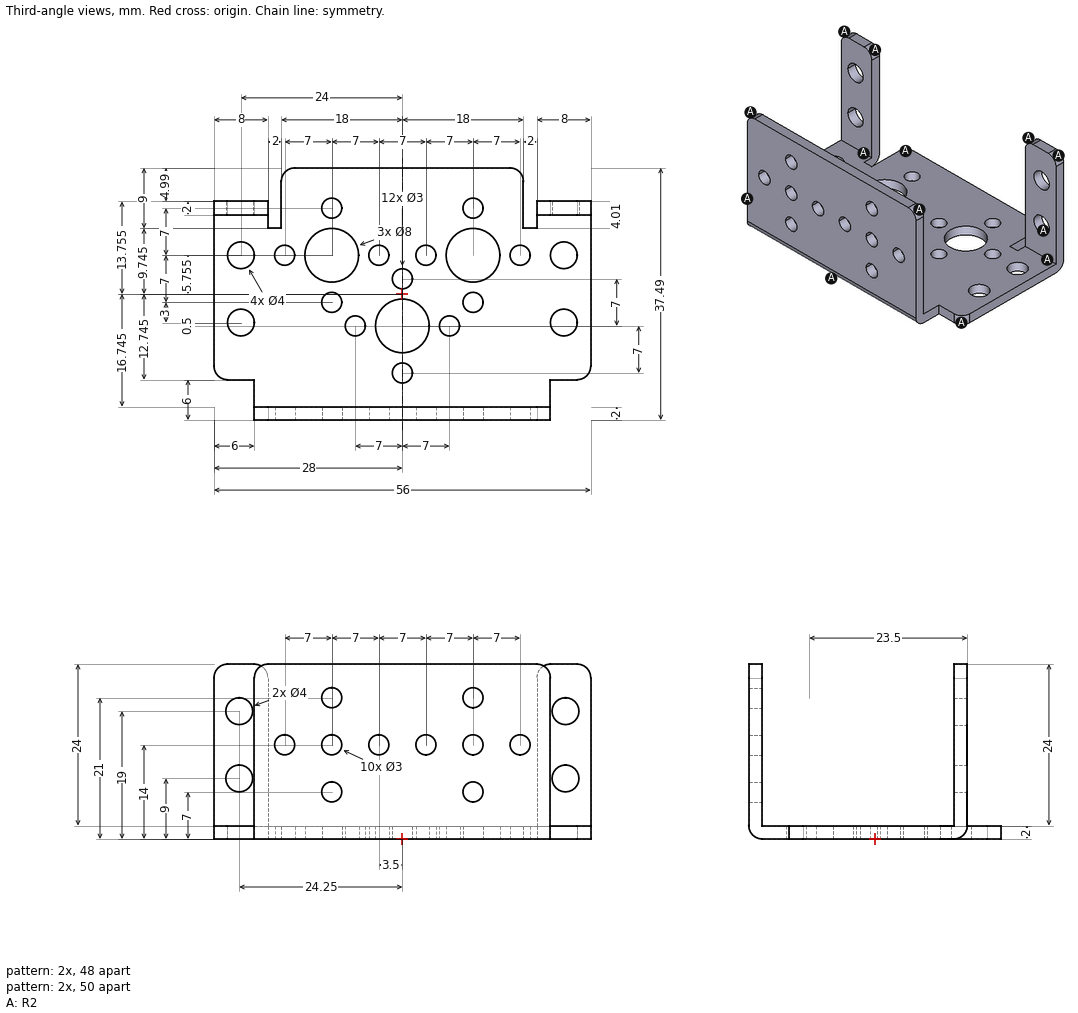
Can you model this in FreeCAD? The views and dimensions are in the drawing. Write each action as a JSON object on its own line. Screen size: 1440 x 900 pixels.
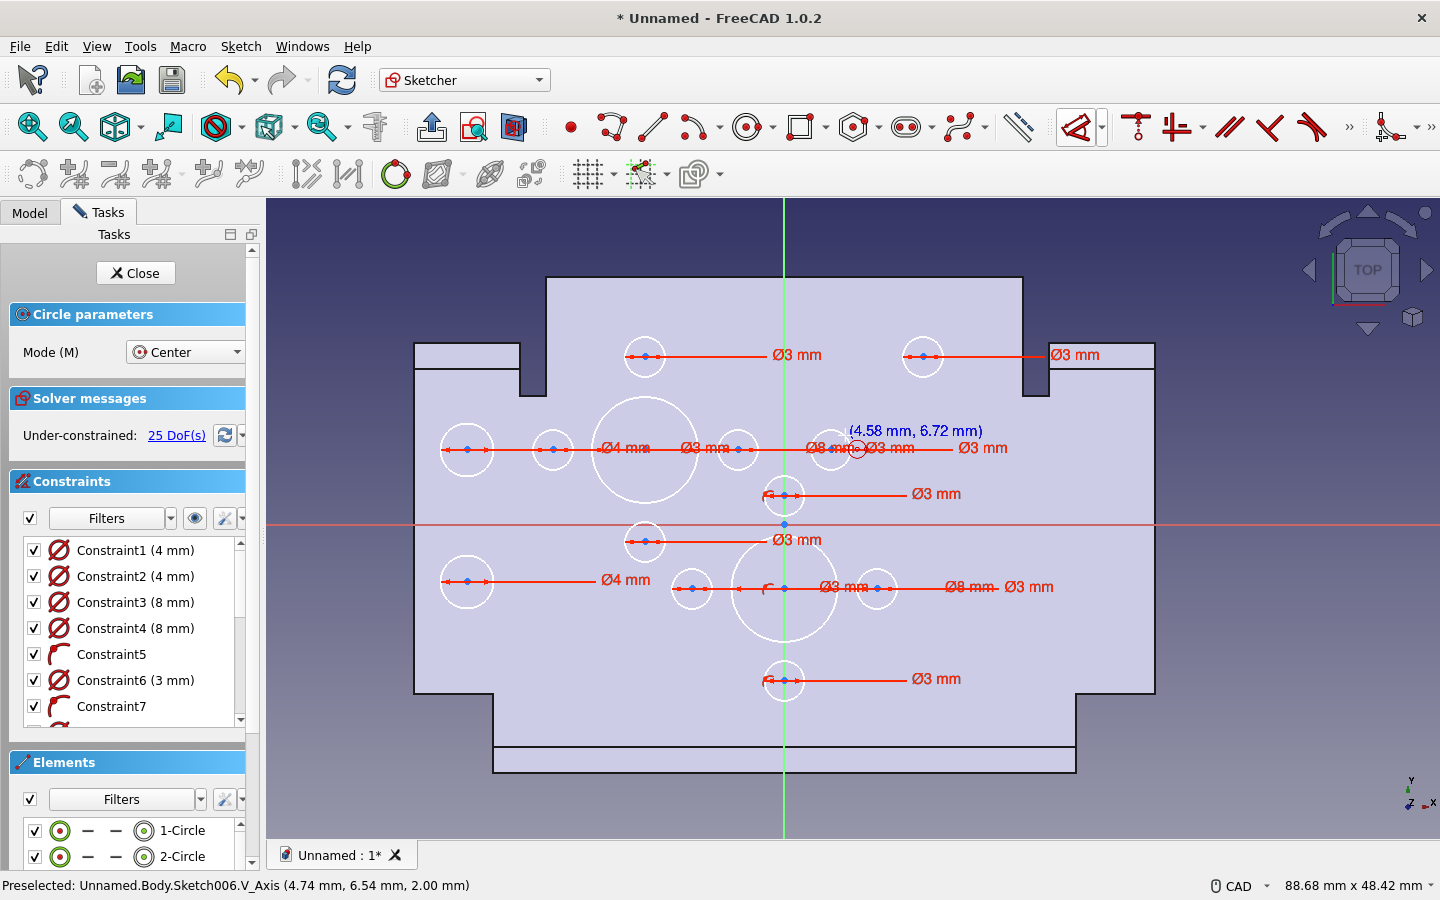
{"action": "left_click", "coordinate": [923, 541]}
{"action": "mouse_move", "coordinate": [937, 555]}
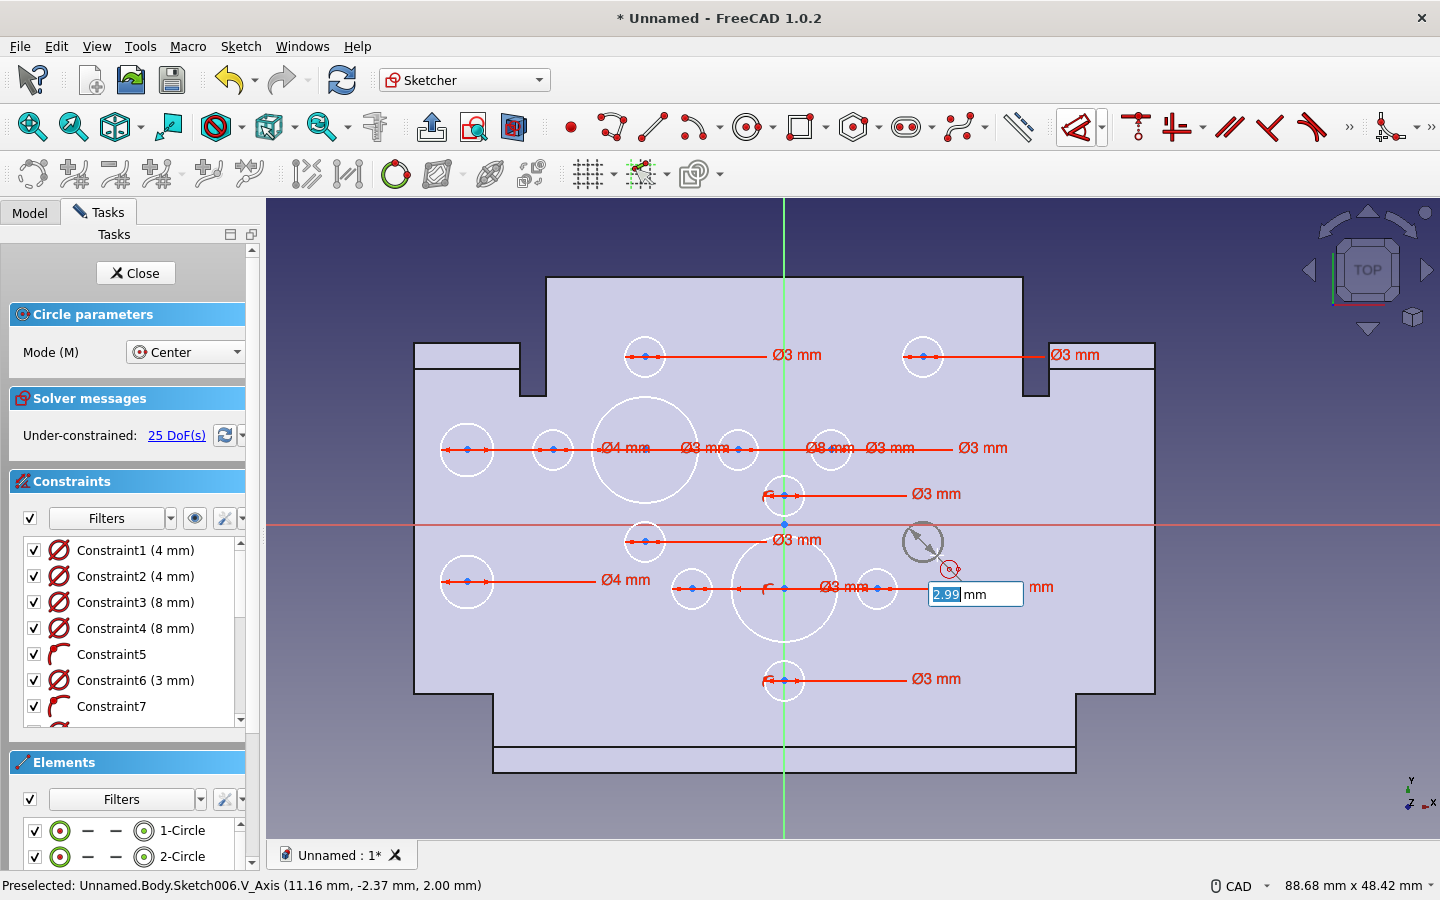
{"action": "type", "text": "3"}
{"action": "key", "text": "Return"}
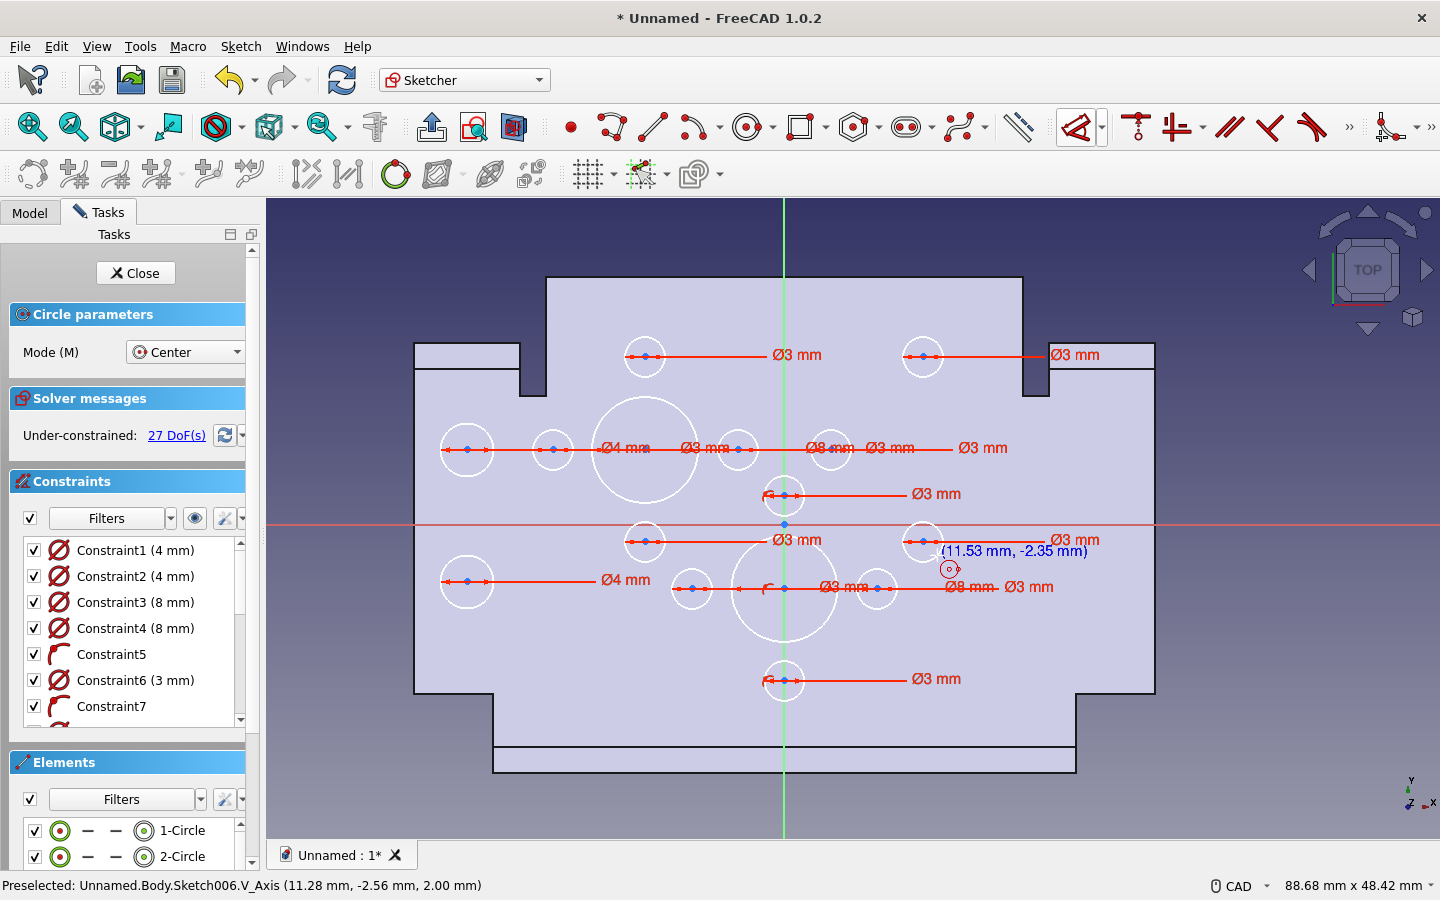
{"action": "left_click", "coordinate": [923, 449]}
{"action": "mouse_move", "coordinate": [961, 411]}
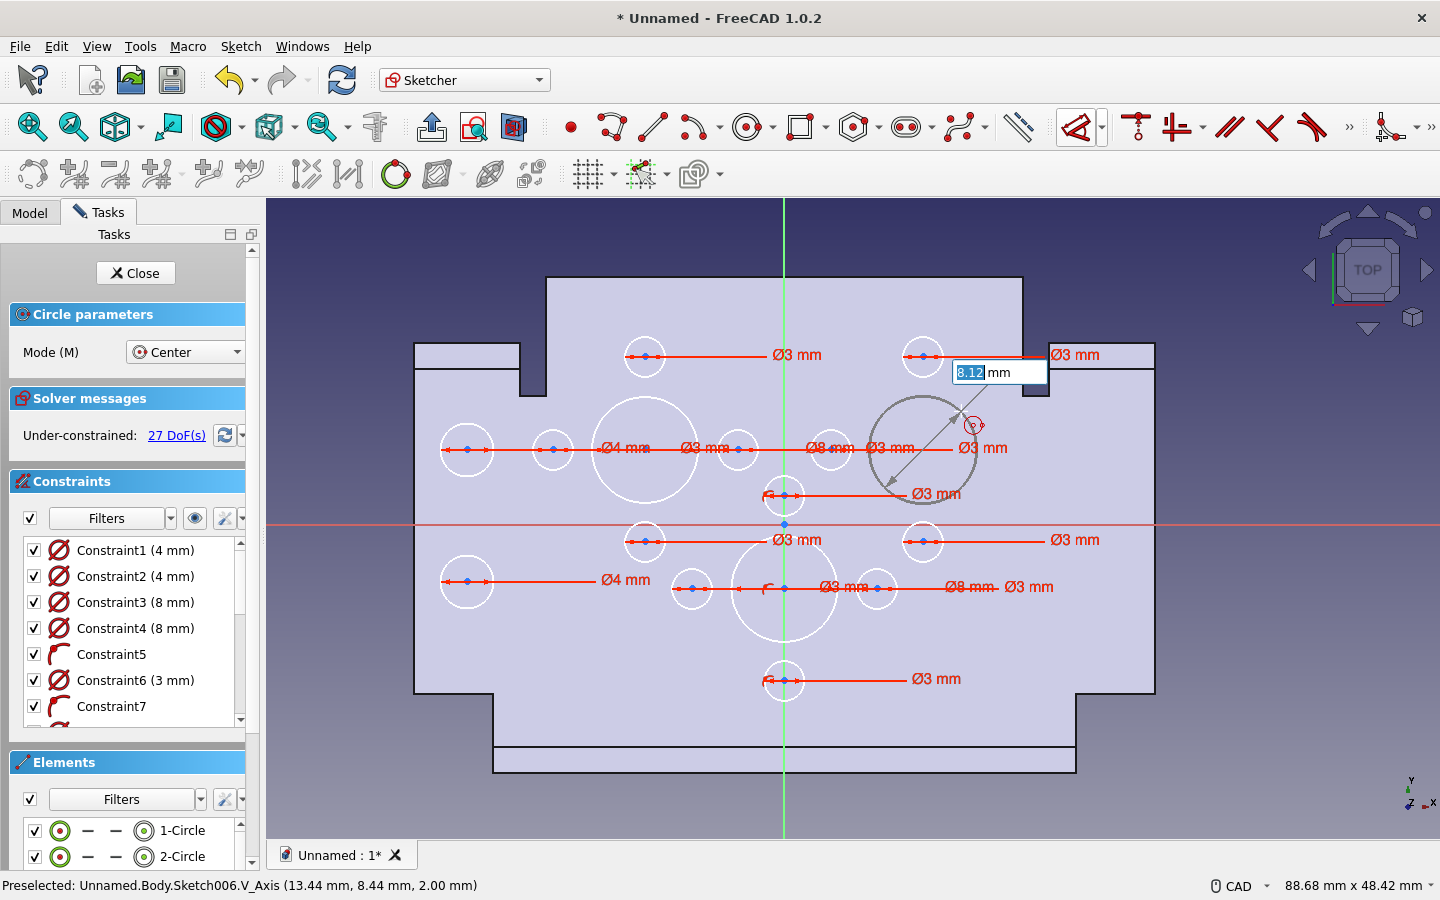
{"action": "type", "text": "8"}
{"action": "key", "text": "Return"}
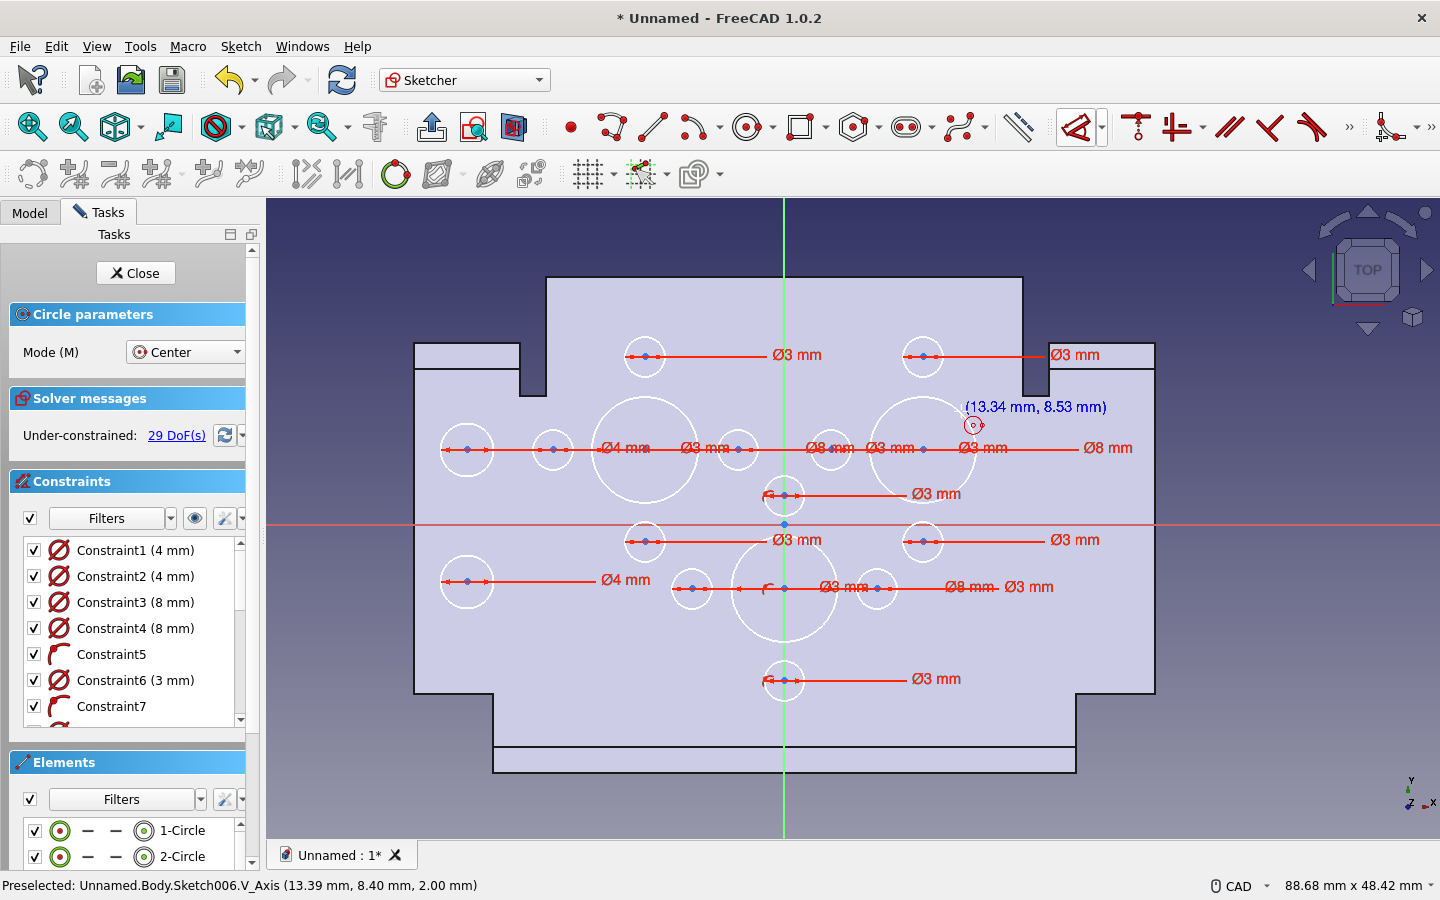
{"action": "left_click", "coordinate": [1016, 449]}
{"action": "mouse_move", "coordinate": [1030, 435]}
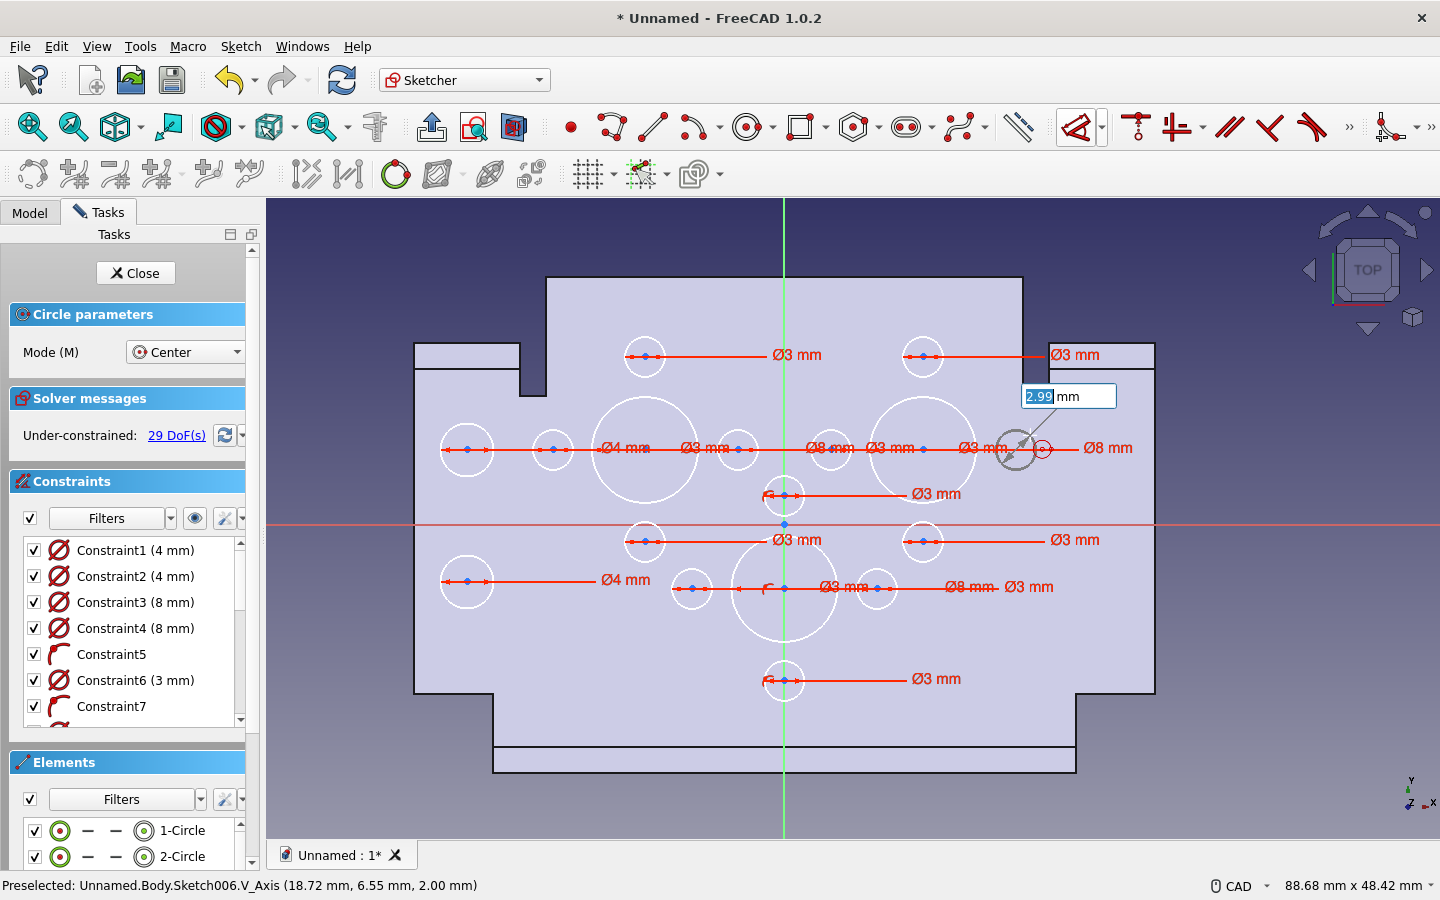
{"action": "type", "text": "3"}
{"action": "key", "text": "Return"}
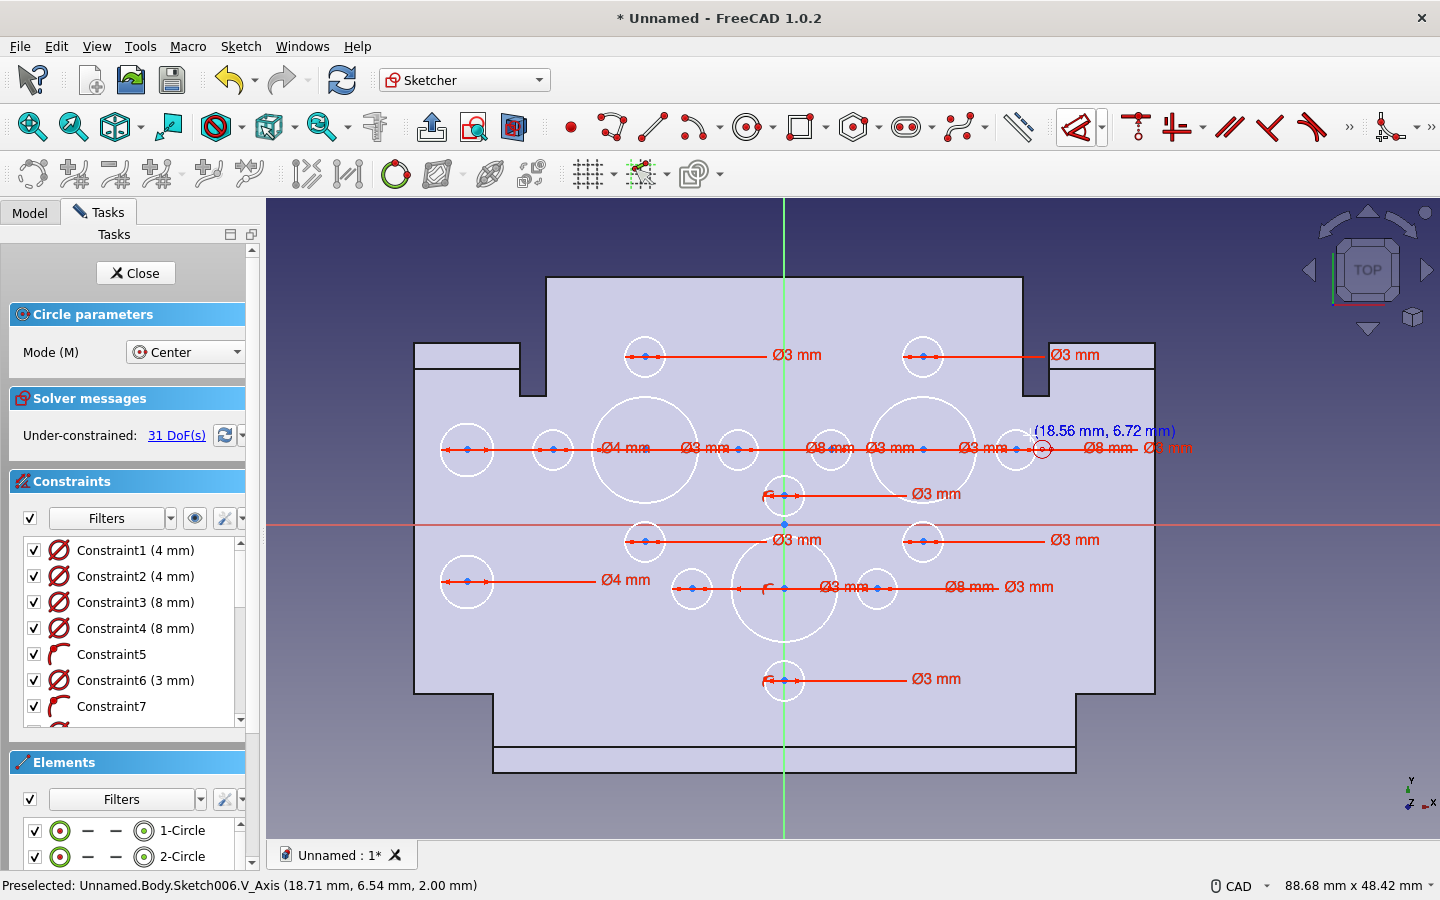
{"action": "left_click", "coordinate": [1102, 581]}
{"action": "mouse_move", "coordinate": [1121, 562]}